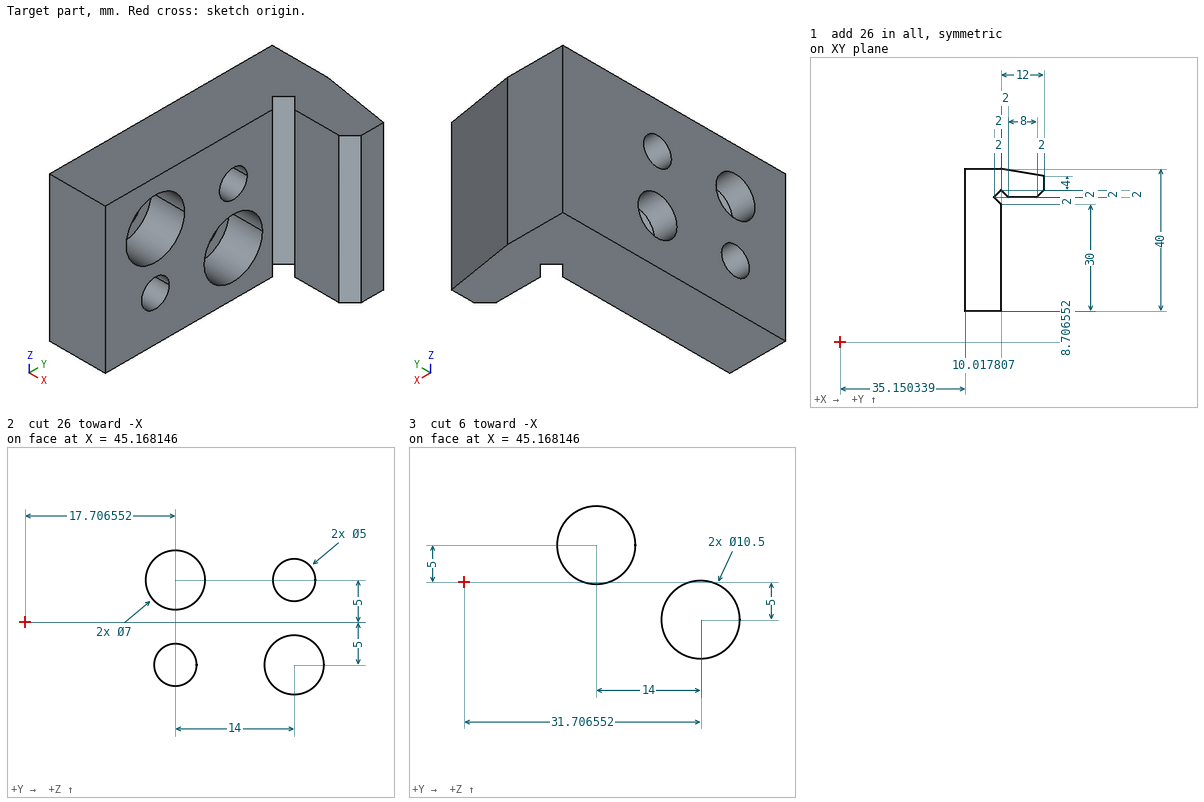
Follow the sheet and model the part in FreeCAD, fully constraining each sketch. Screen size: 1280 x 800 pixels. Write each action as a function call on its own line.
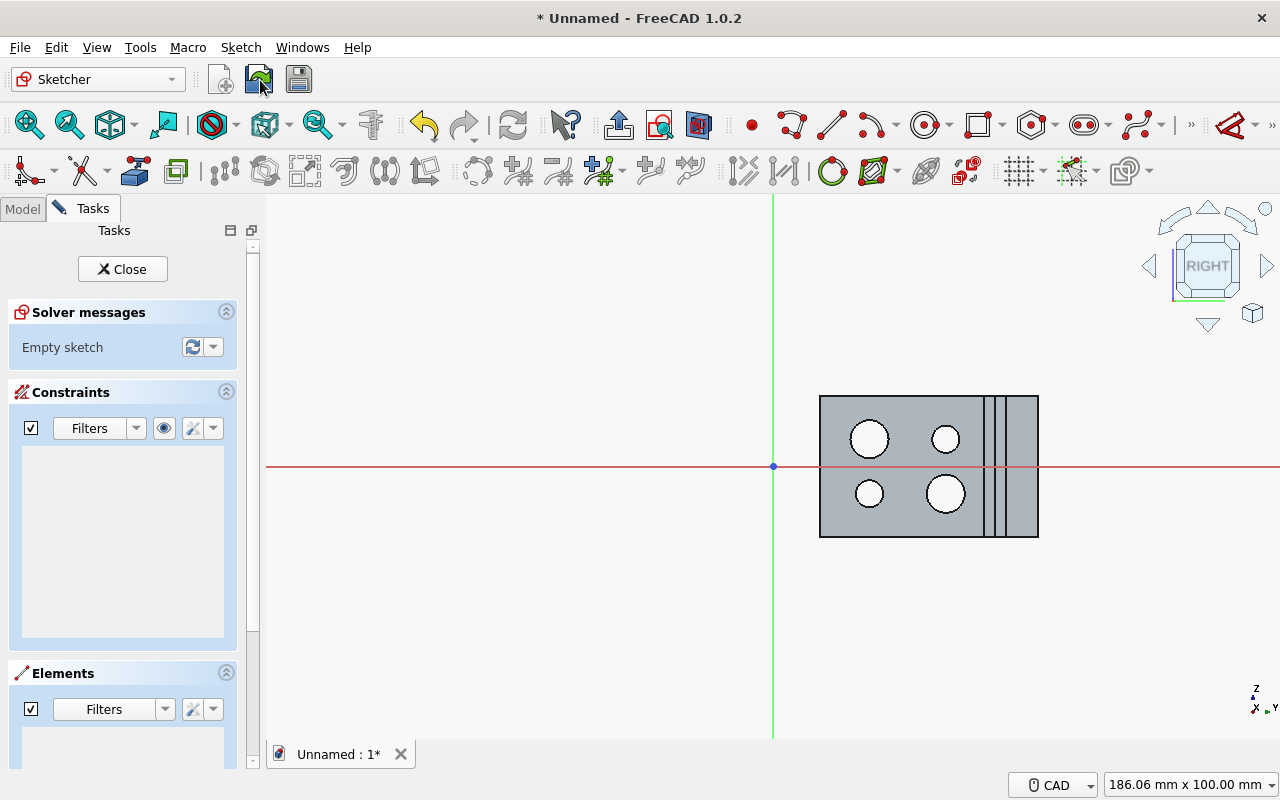
scroll(972, 466, up, 5)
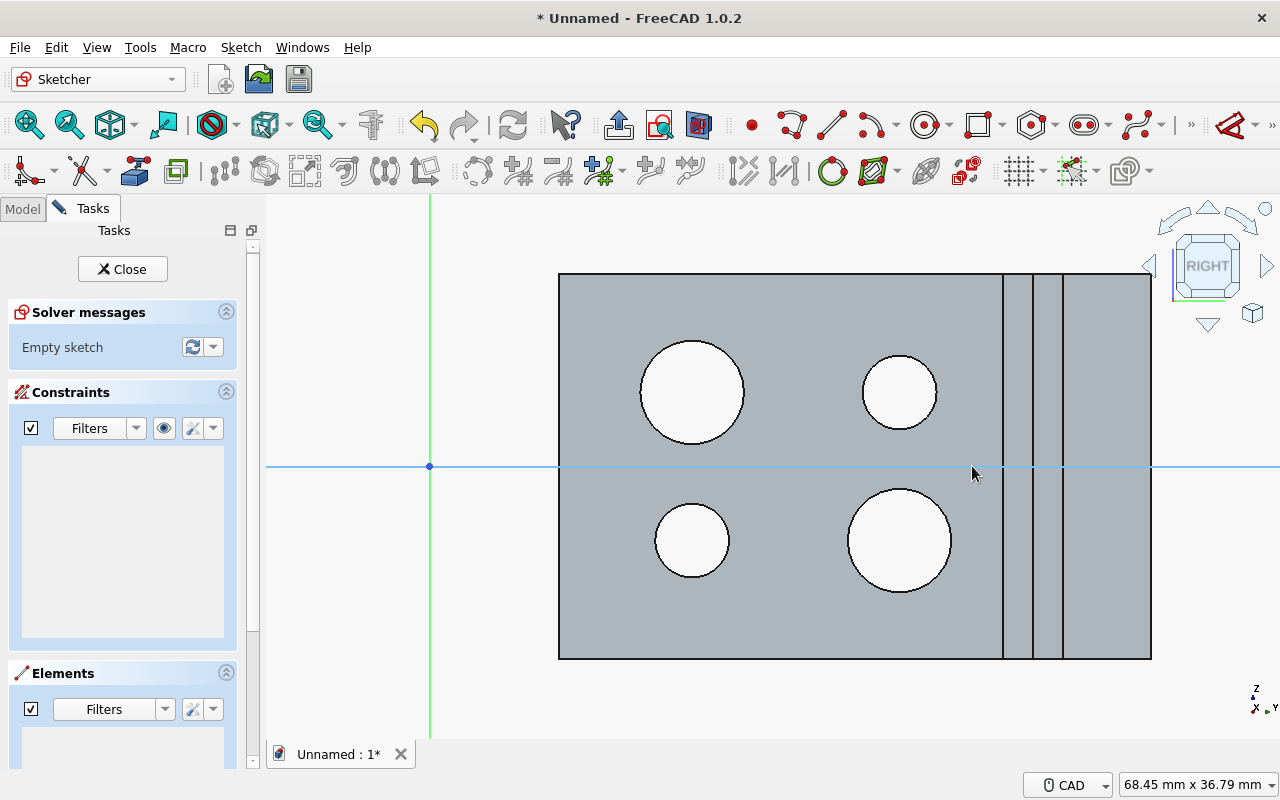
key(g)
key(c)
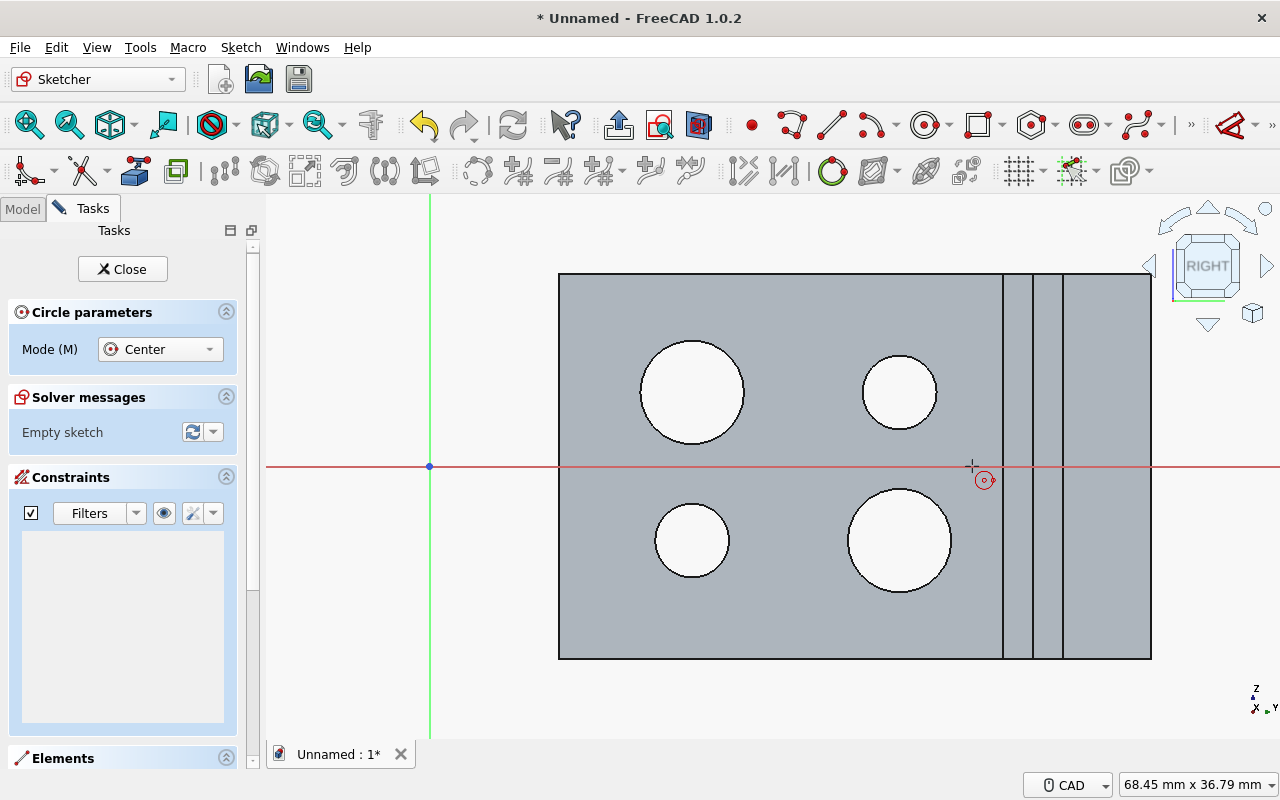
click(900, 541)
move(955, 486)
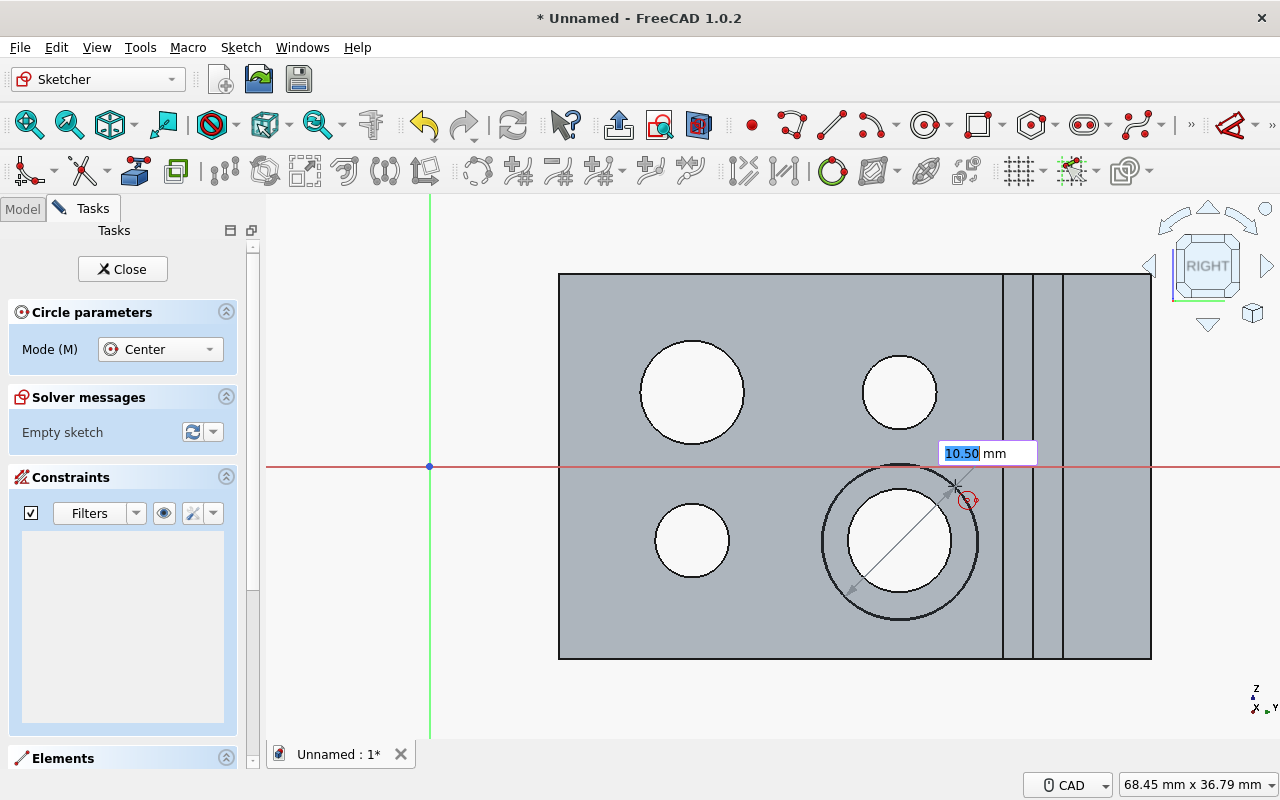
text(10.5)
key(Return)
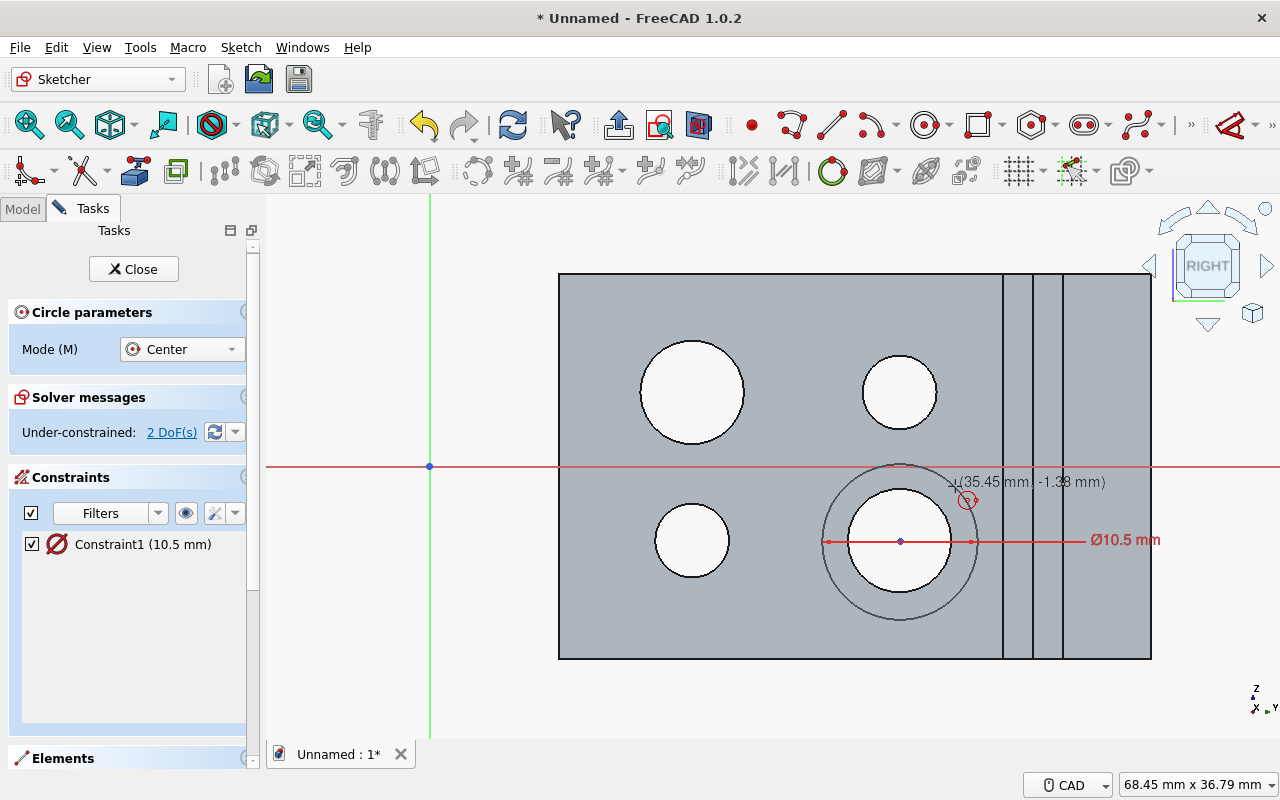
click(692, 392)
move(747, 337)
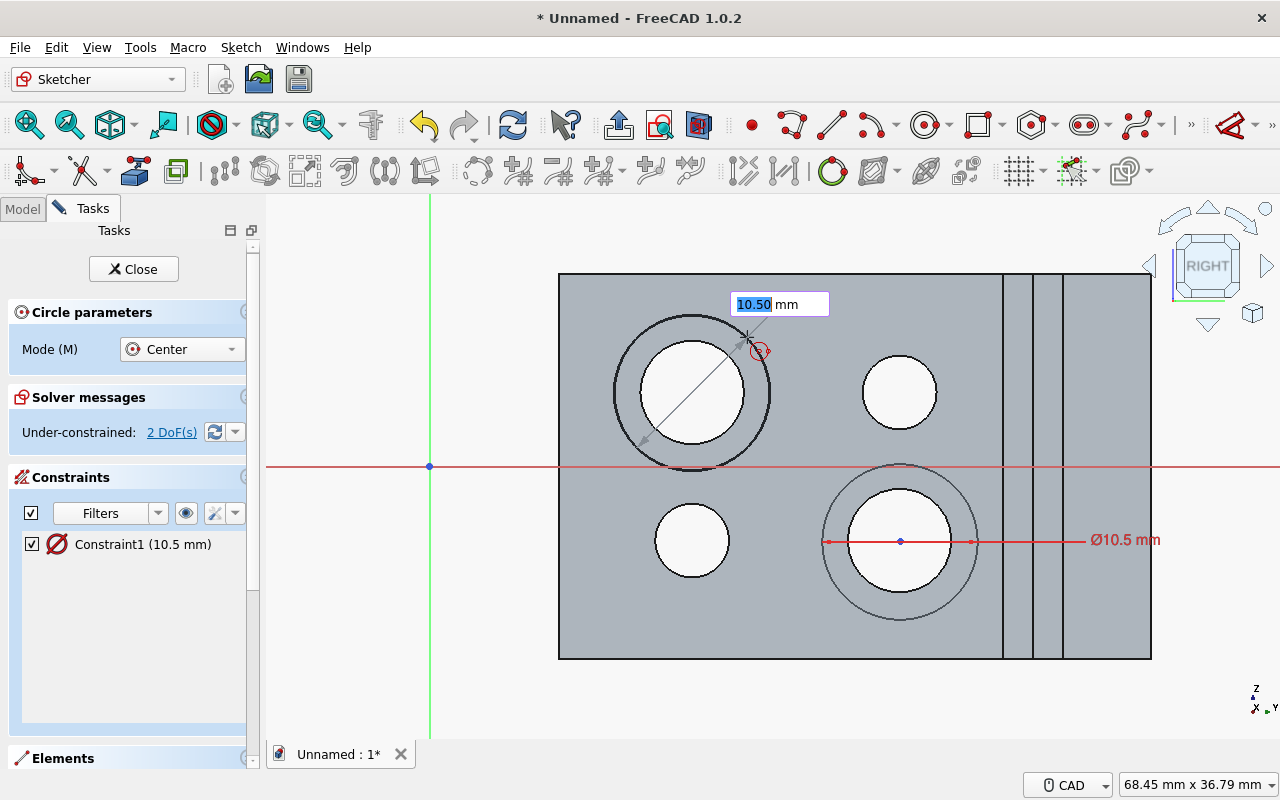
text(10.5)
key(Return)
key(Escape)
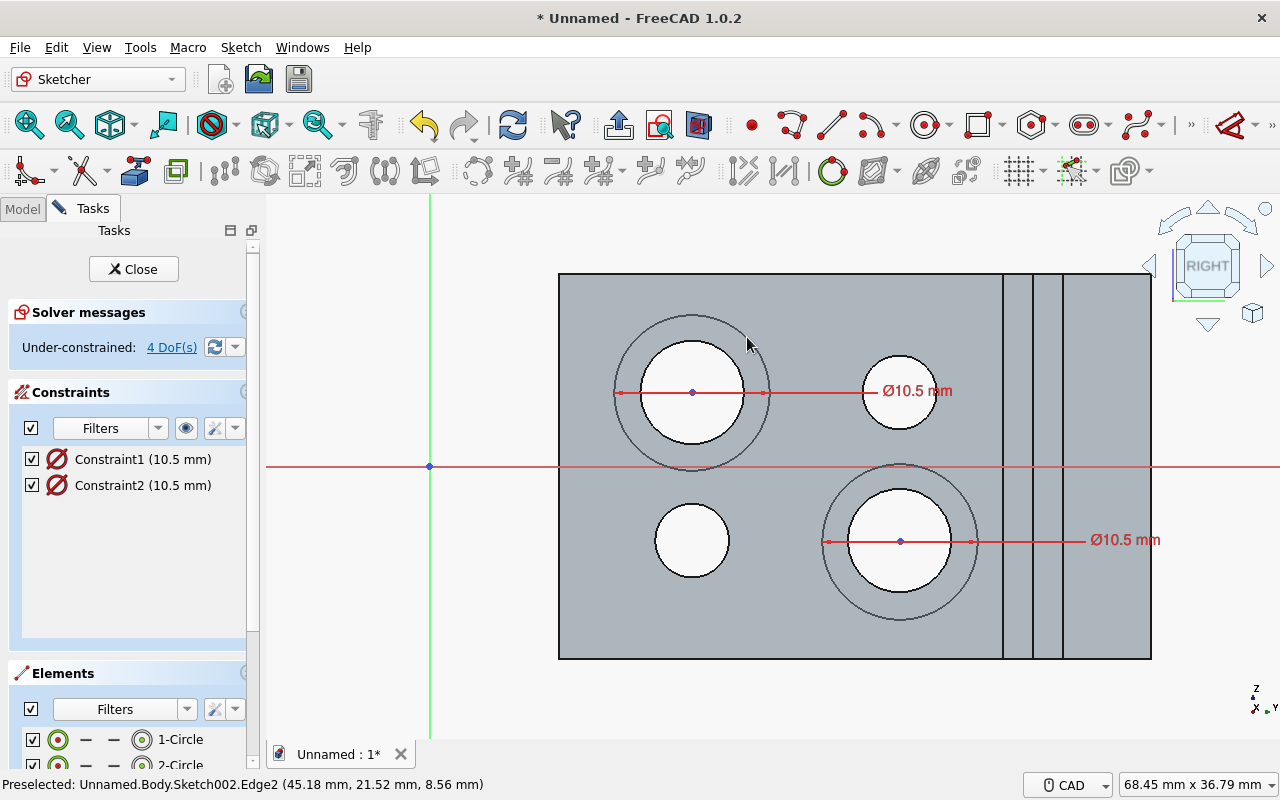
key(d)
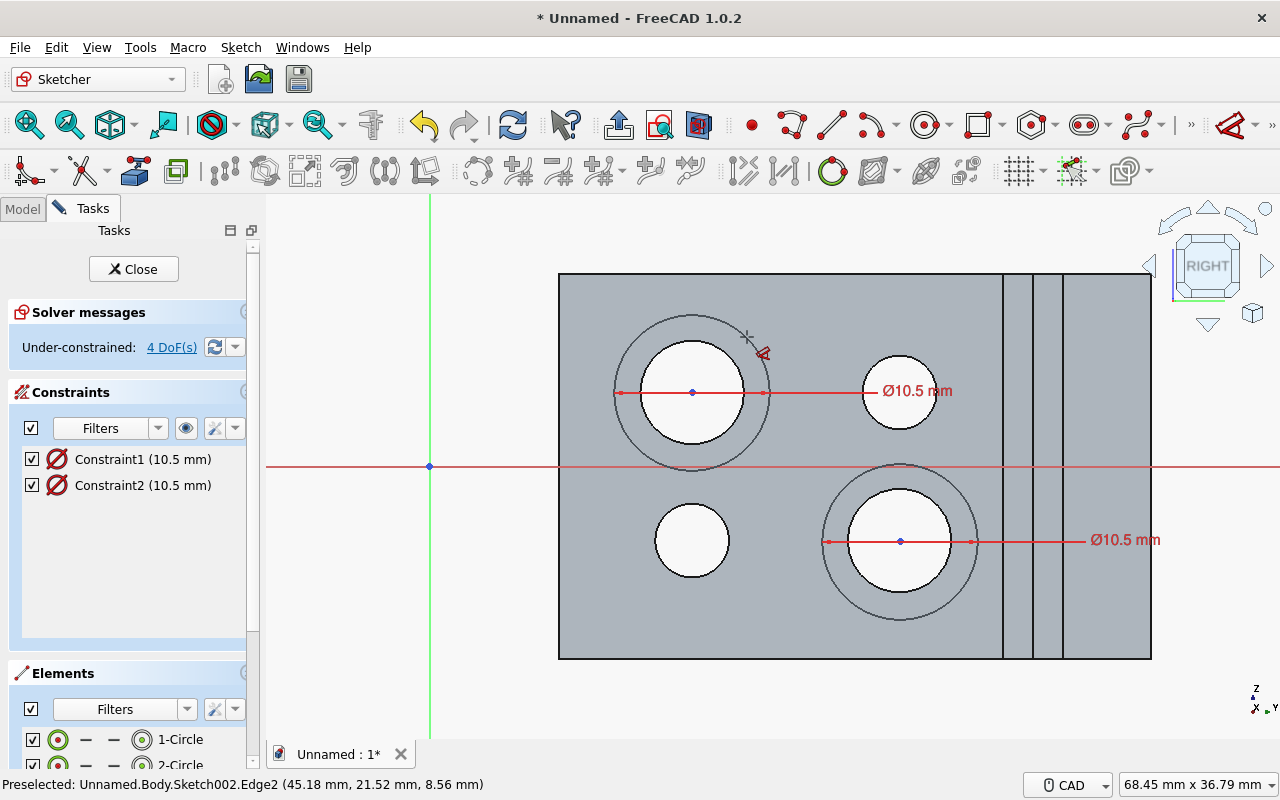
click(900, 542)
click(396, 504)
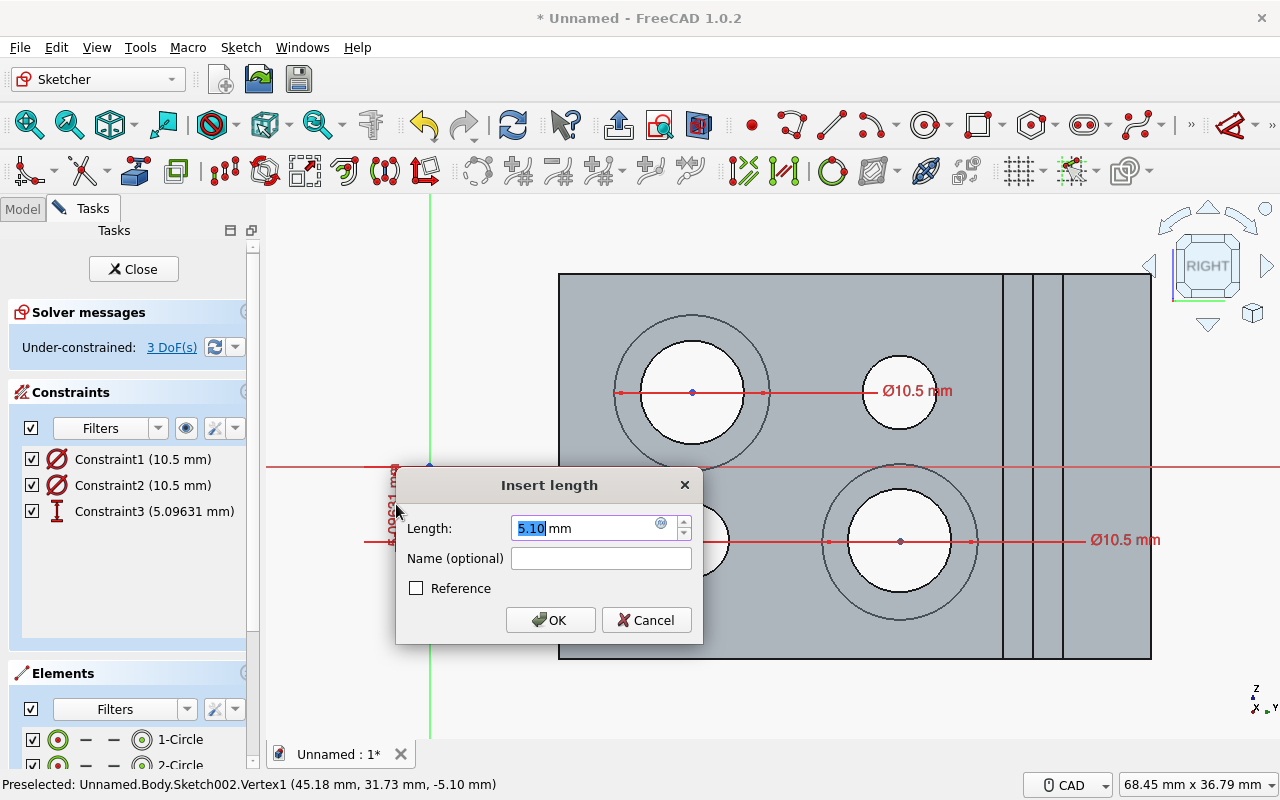
text(5)
key(Return)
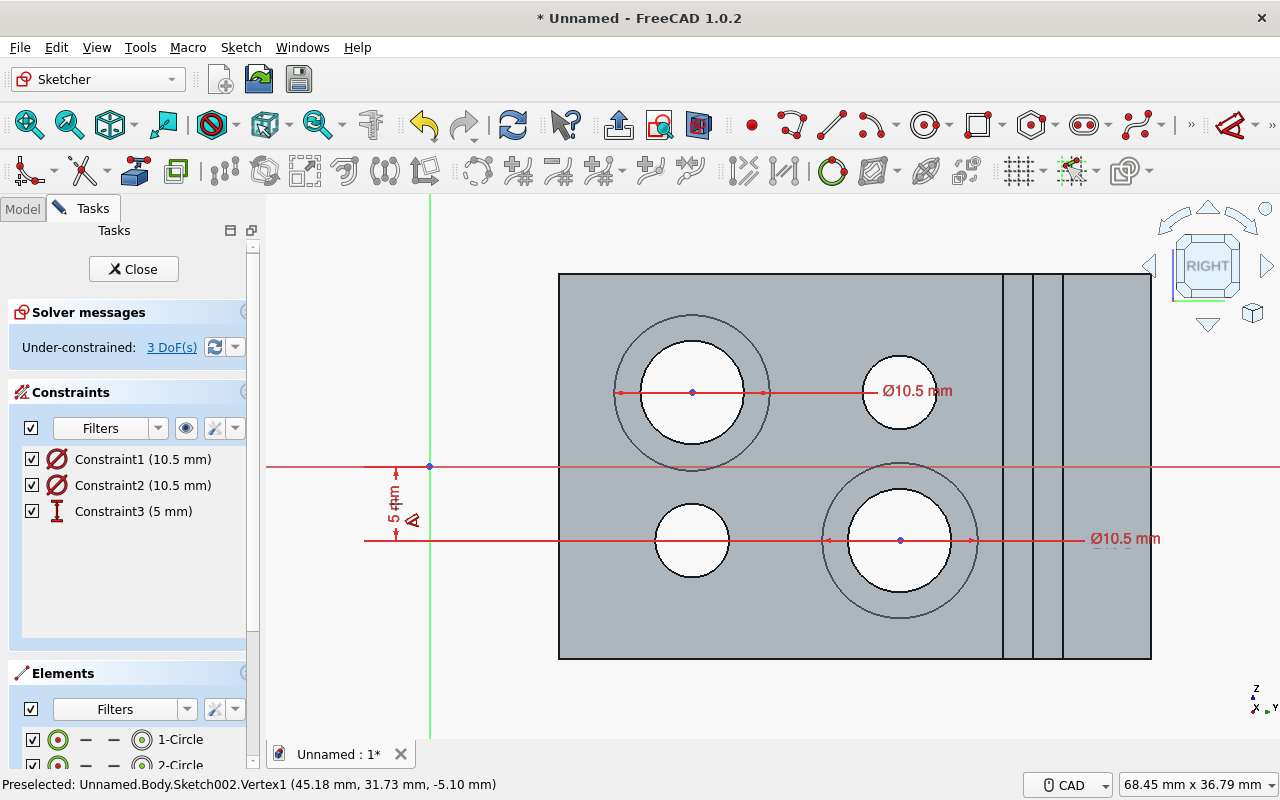
click(692, 393)
click(396, 430)